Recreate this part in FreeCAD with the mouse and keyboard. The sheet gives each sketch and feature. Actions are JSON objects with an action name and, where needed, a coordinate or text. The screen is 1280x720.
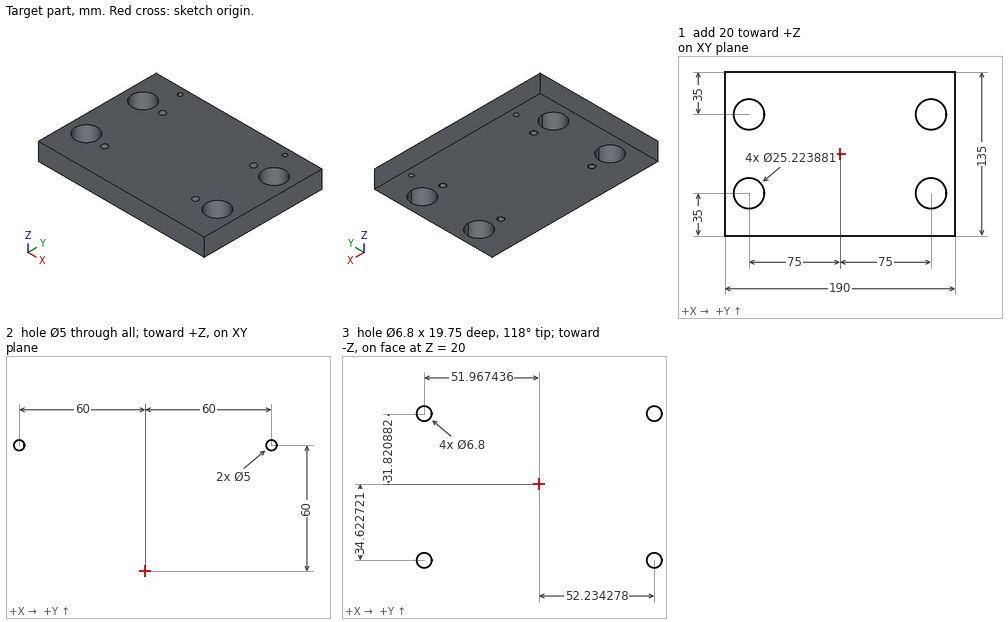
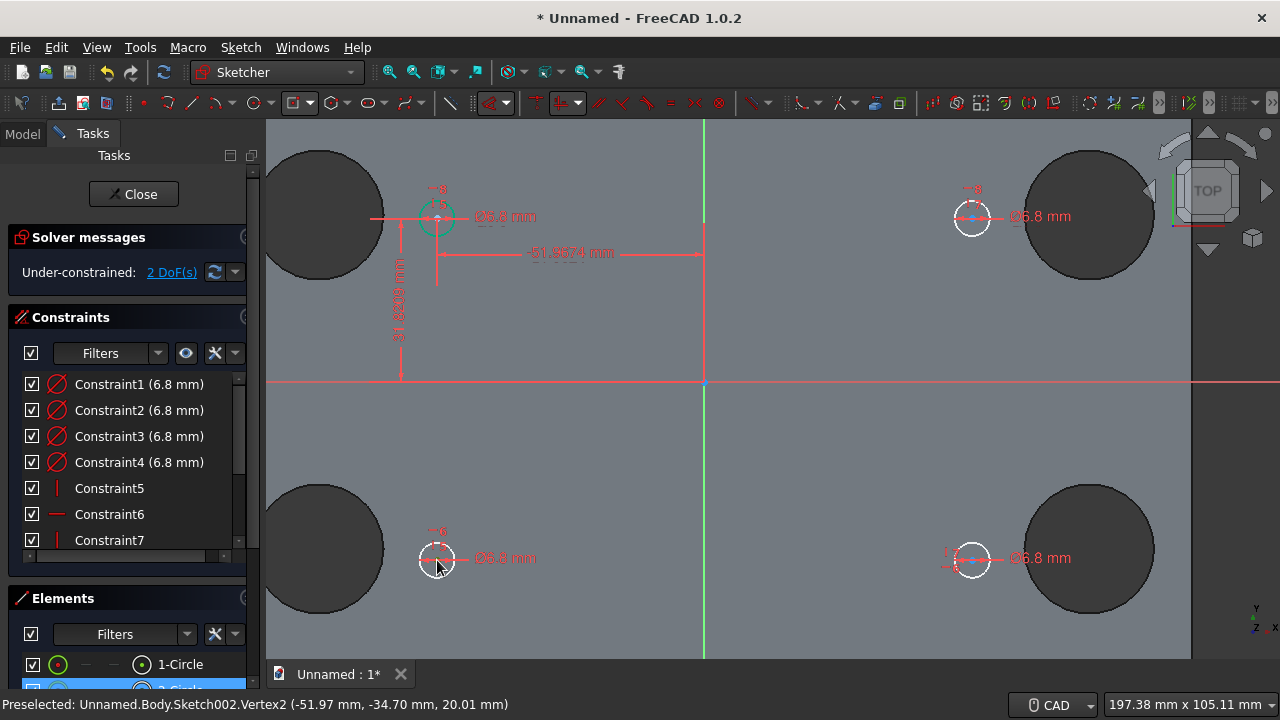
{"action": "key", "text": "i"}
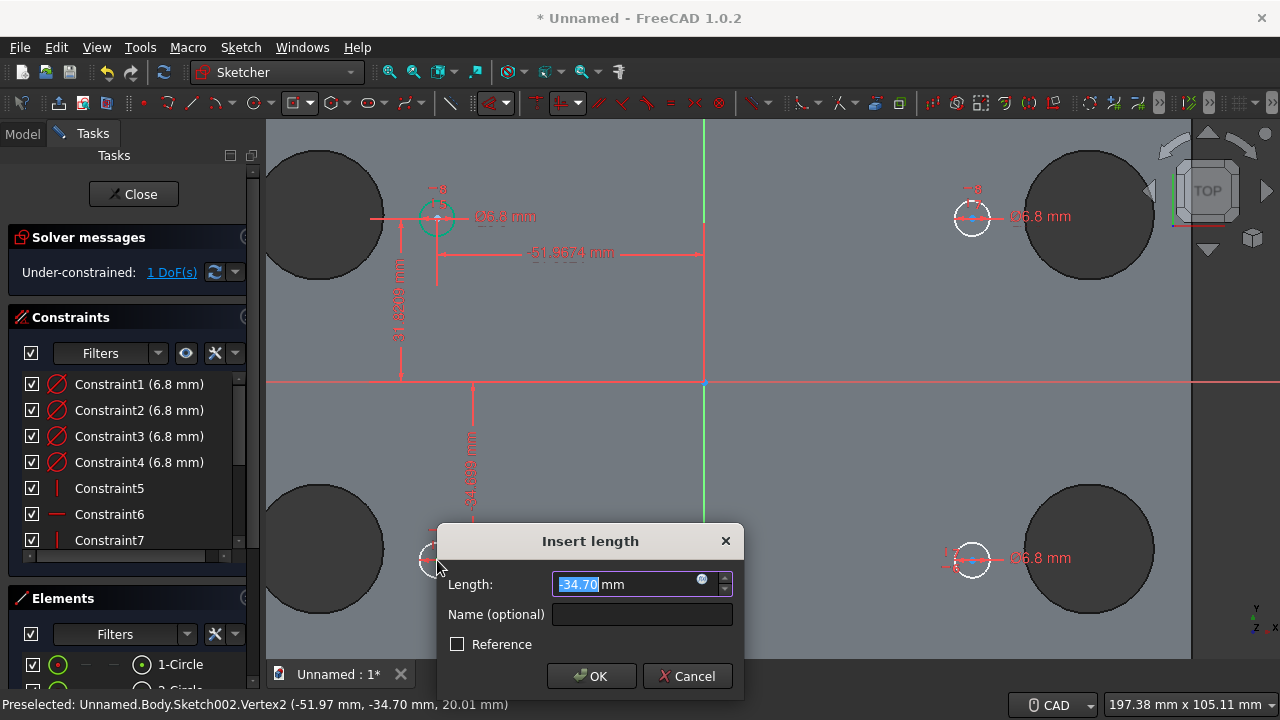
{"action": "type", "text": "-34.622721"}
{"action": "key", "text": "Return"}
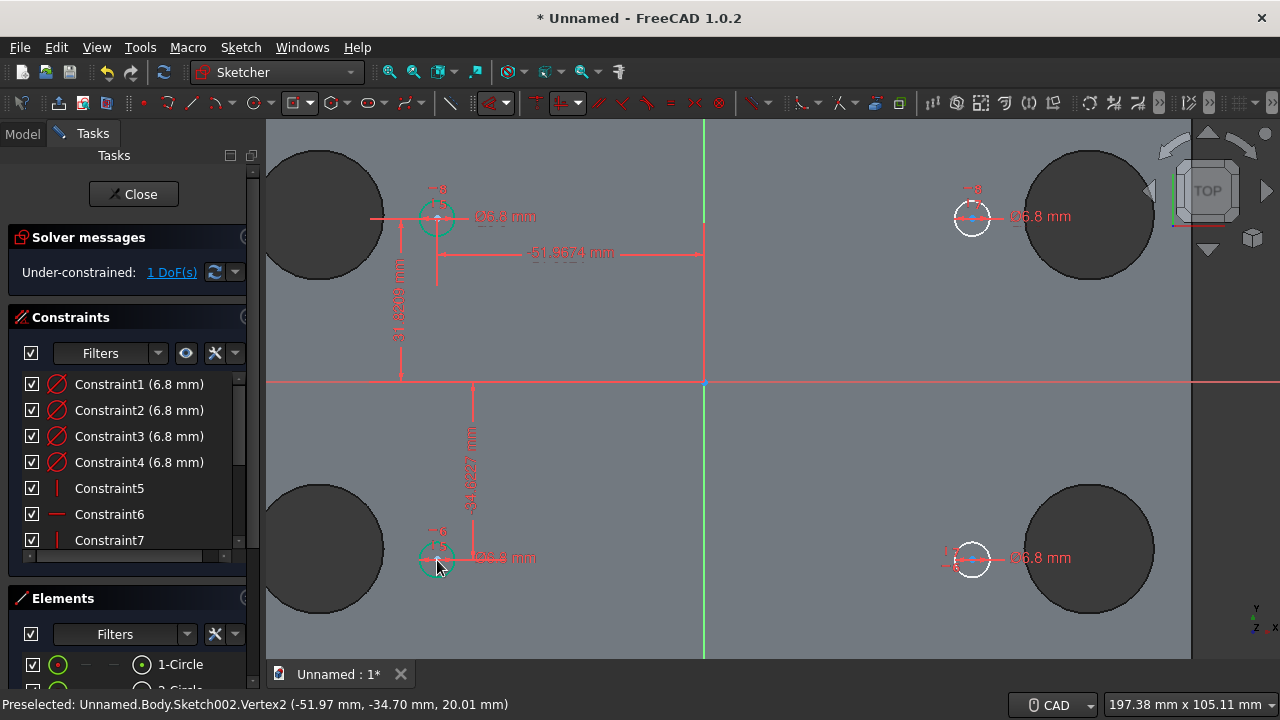
{"action": "left_click", "coordinate": [972, 560]}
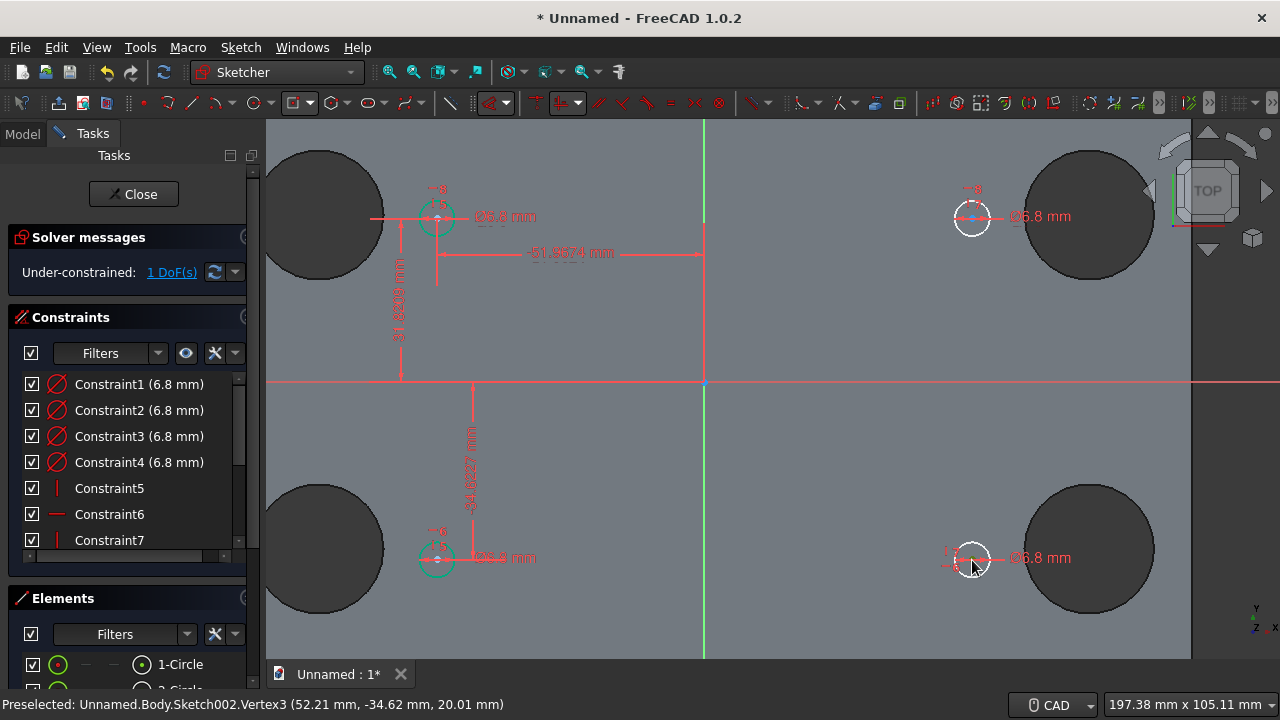
{"action": "key", "text": "l"}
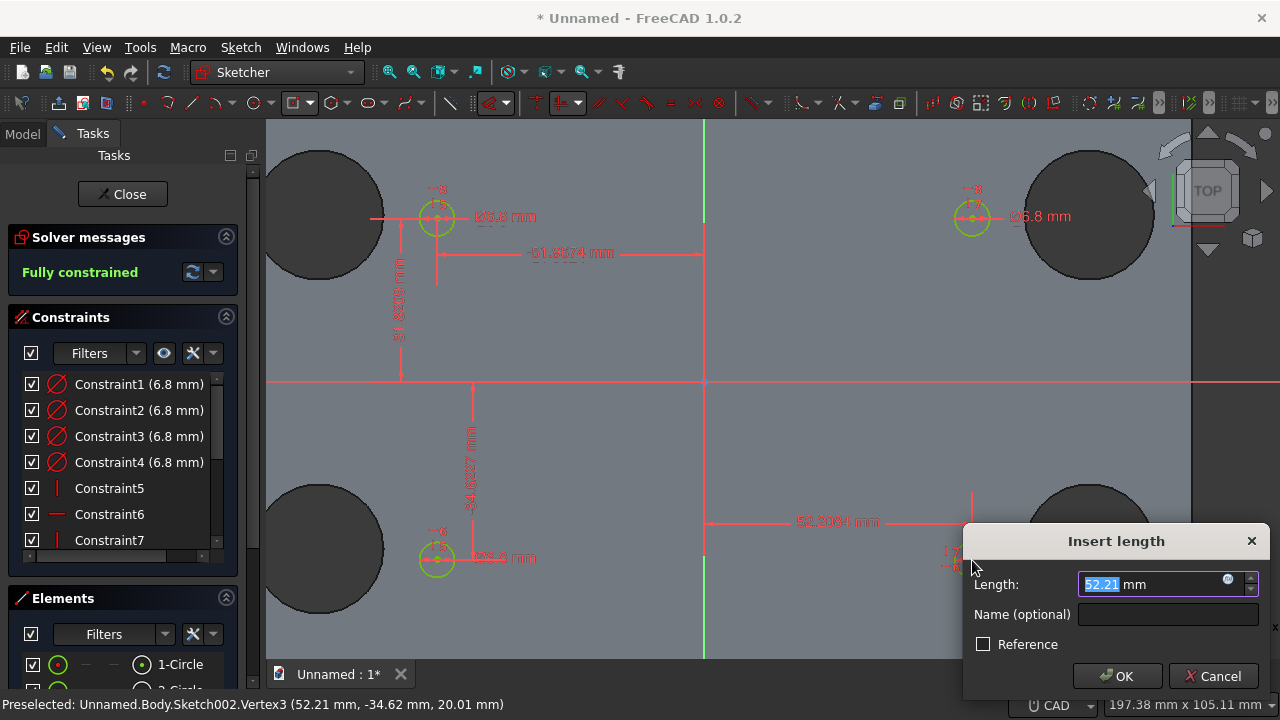
{"action": "type", "text": "52.234278"}
{"action": "key", "text": "Return"}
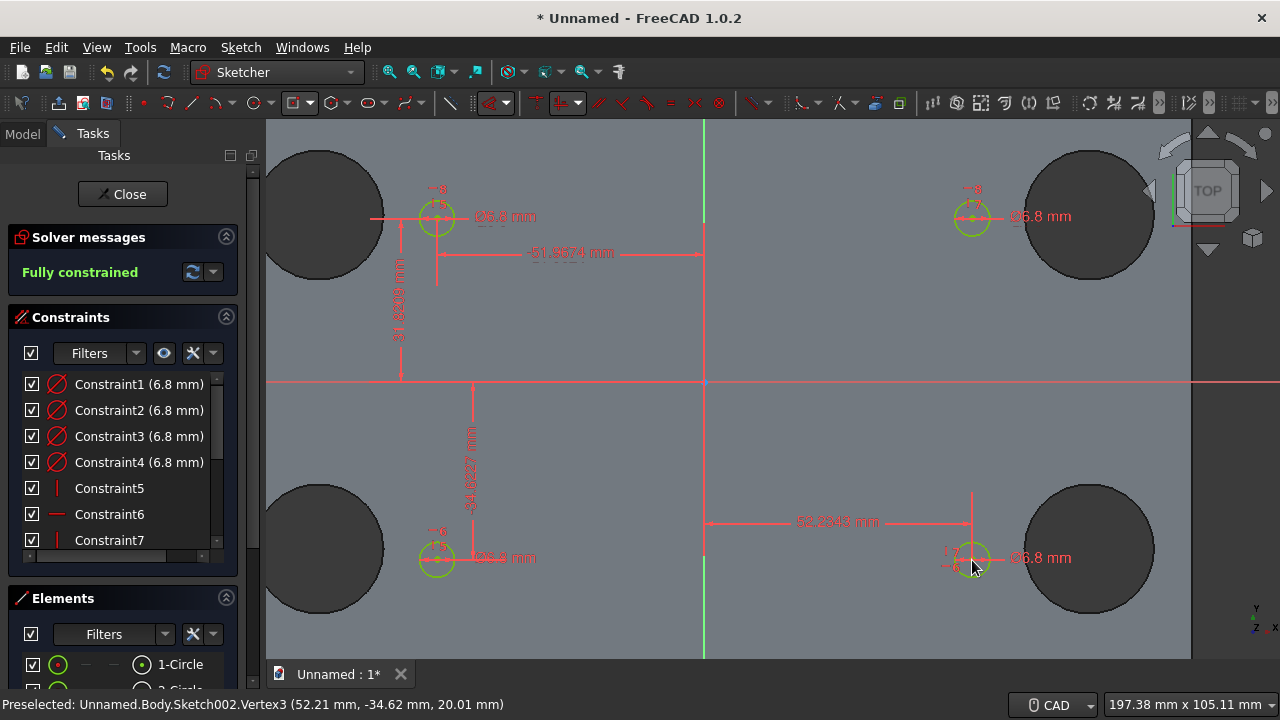
{"action": "left_click", "coordinate": [123, 194]}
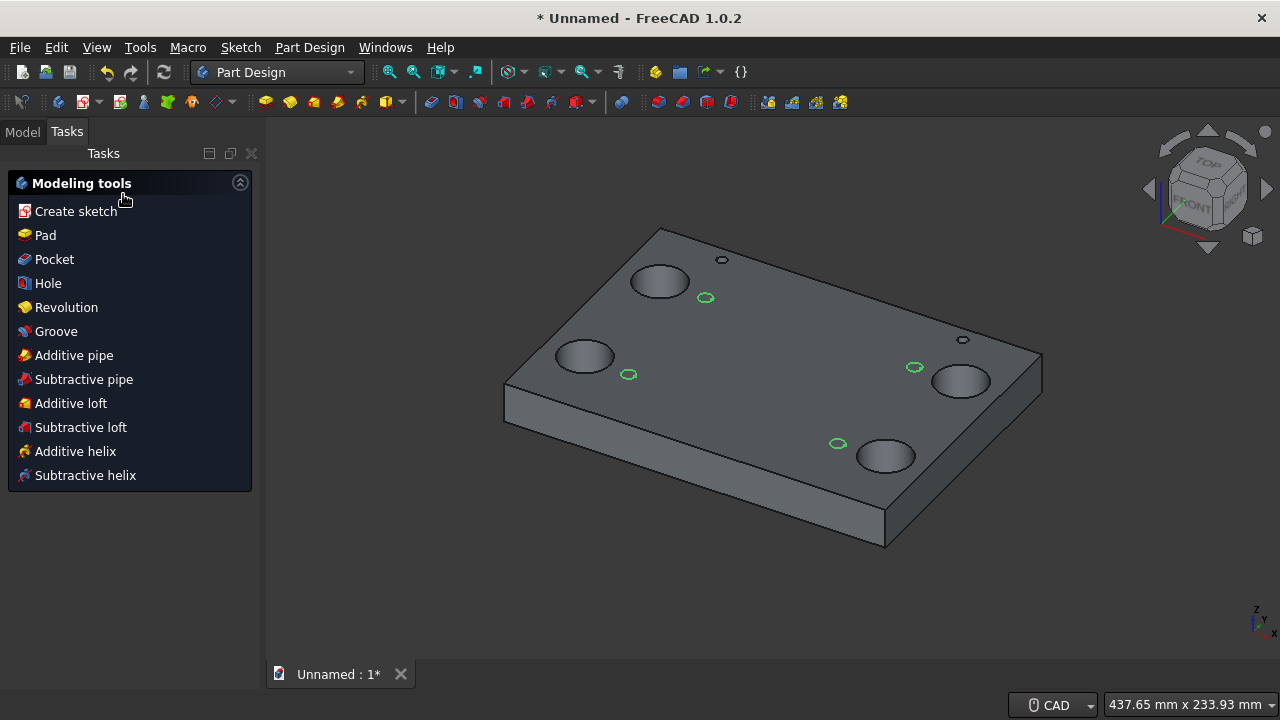
{"action": "left_click", "coordinate": [456, 102]}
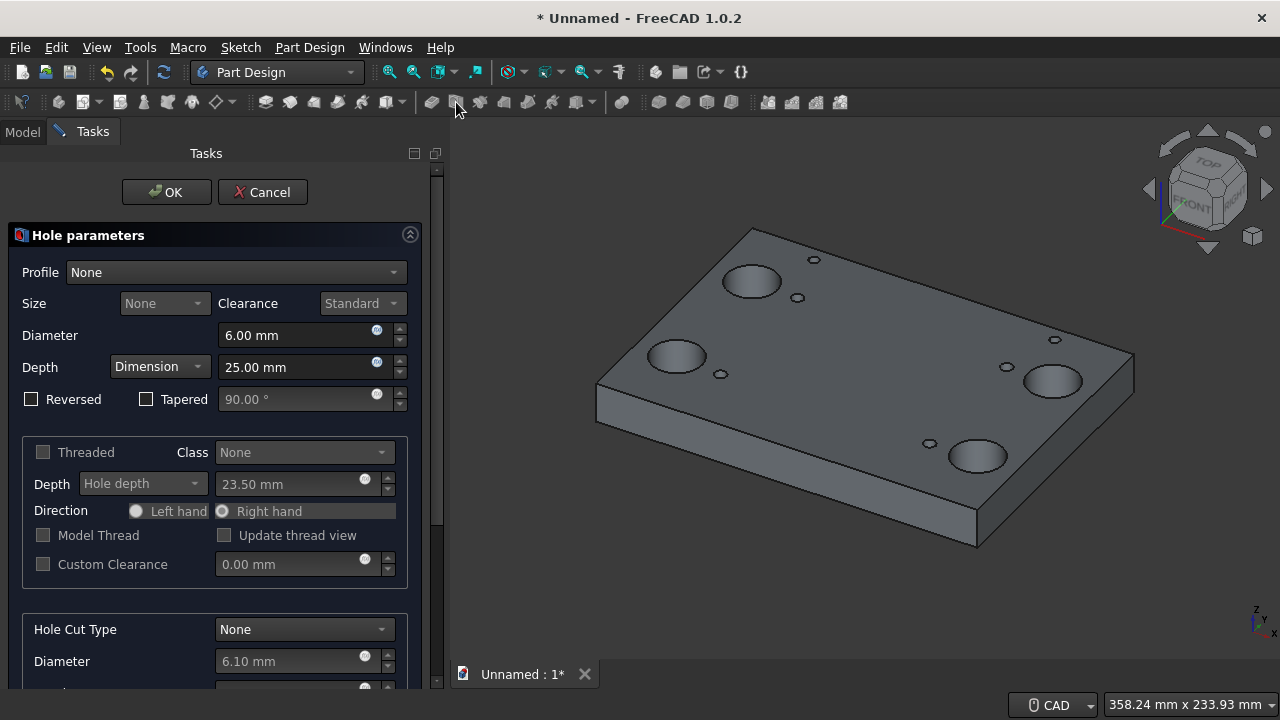
{"action": "triple_click", "coordinate": [305, 335]}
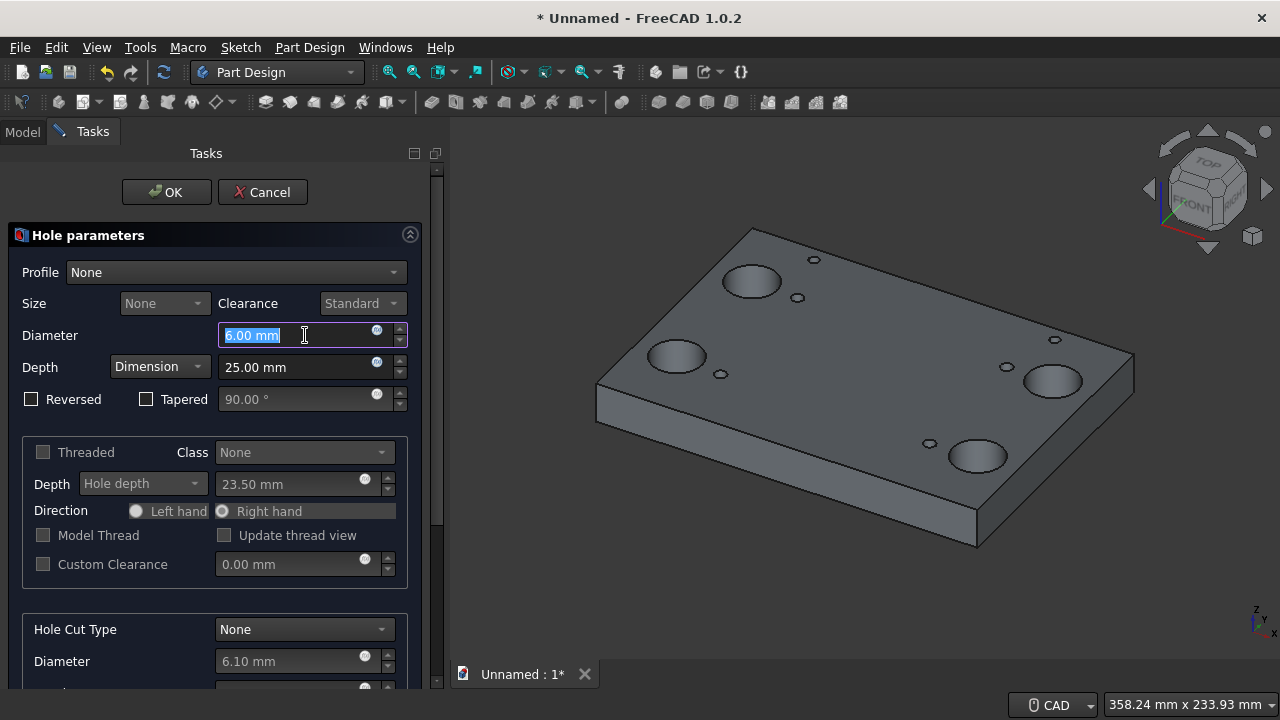
{"action": "type", "text": "6.8"}
{"action": "key", "text": "Tab"}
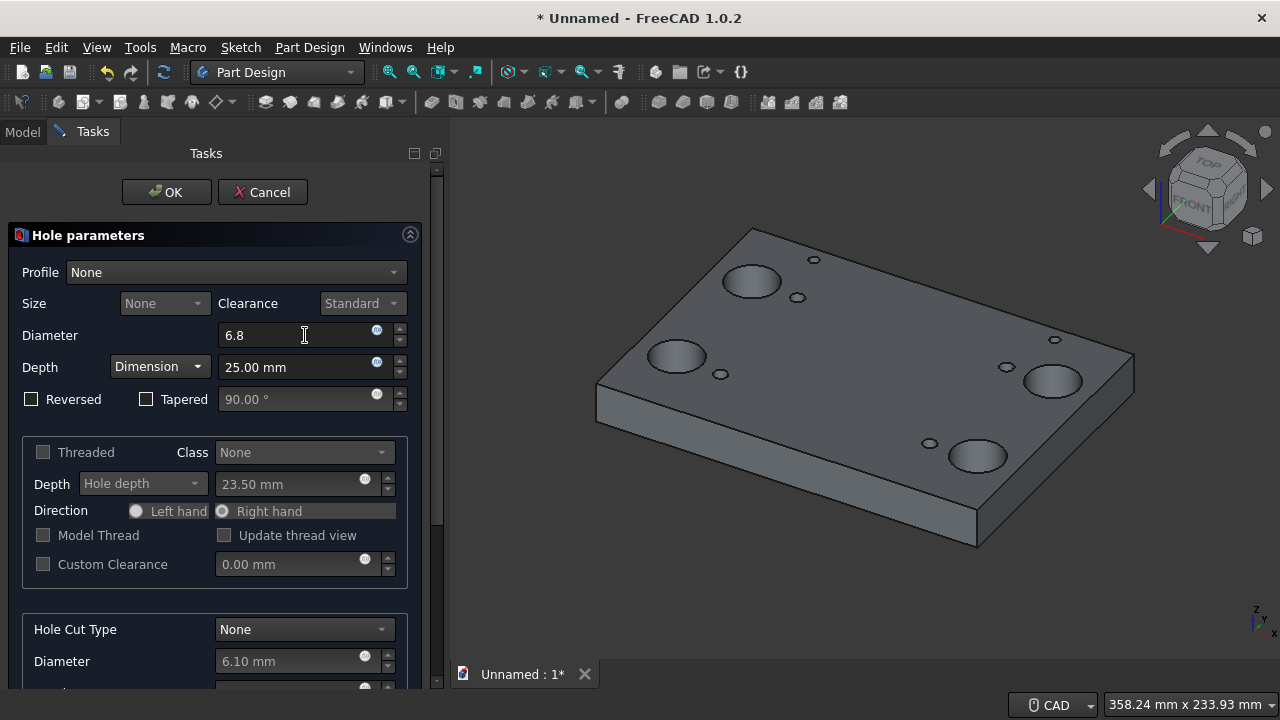
{"action": "triple_click", "coordinate": [305, 367]}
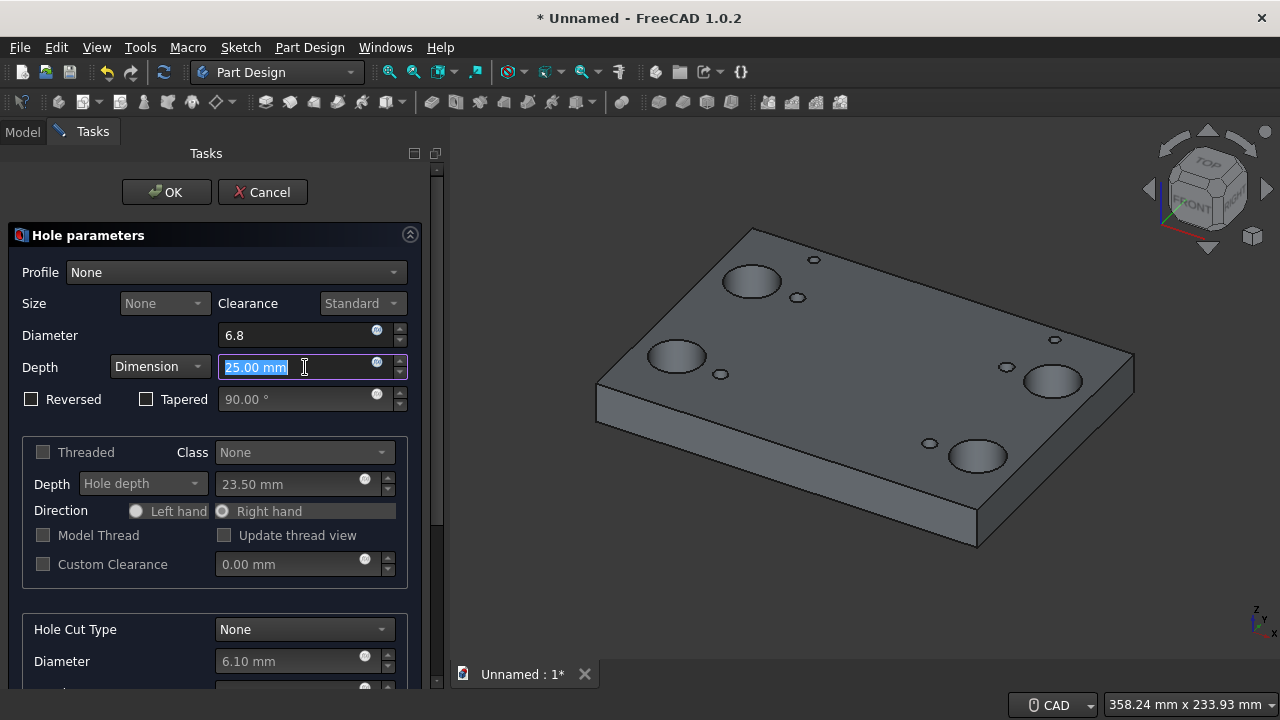
{"action": "type", "text": "19.75"}
{"action": "key", "text": "Tab"}